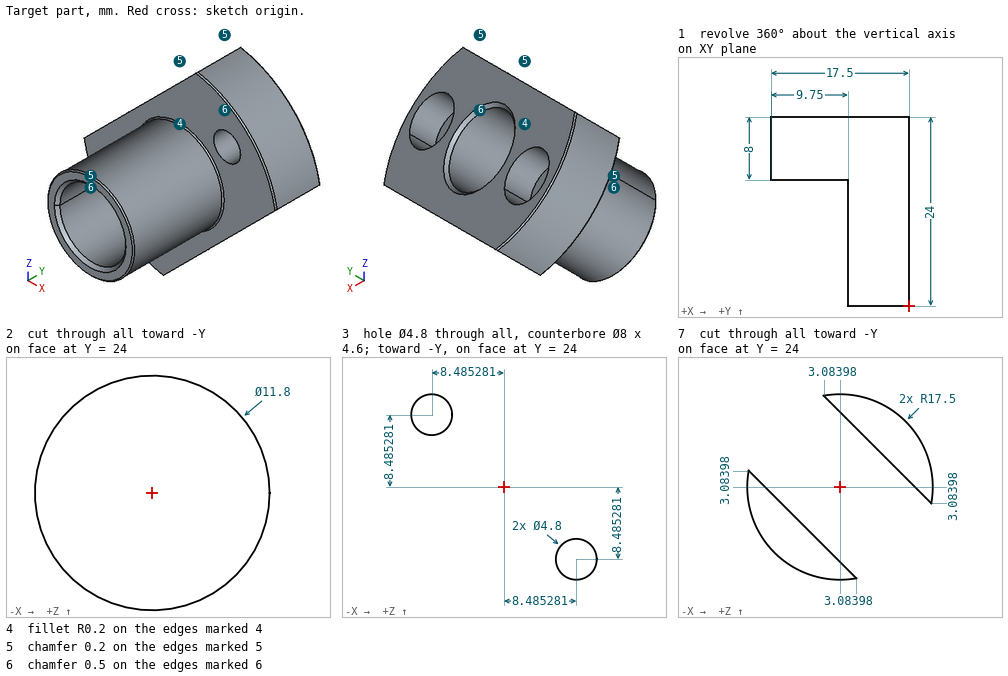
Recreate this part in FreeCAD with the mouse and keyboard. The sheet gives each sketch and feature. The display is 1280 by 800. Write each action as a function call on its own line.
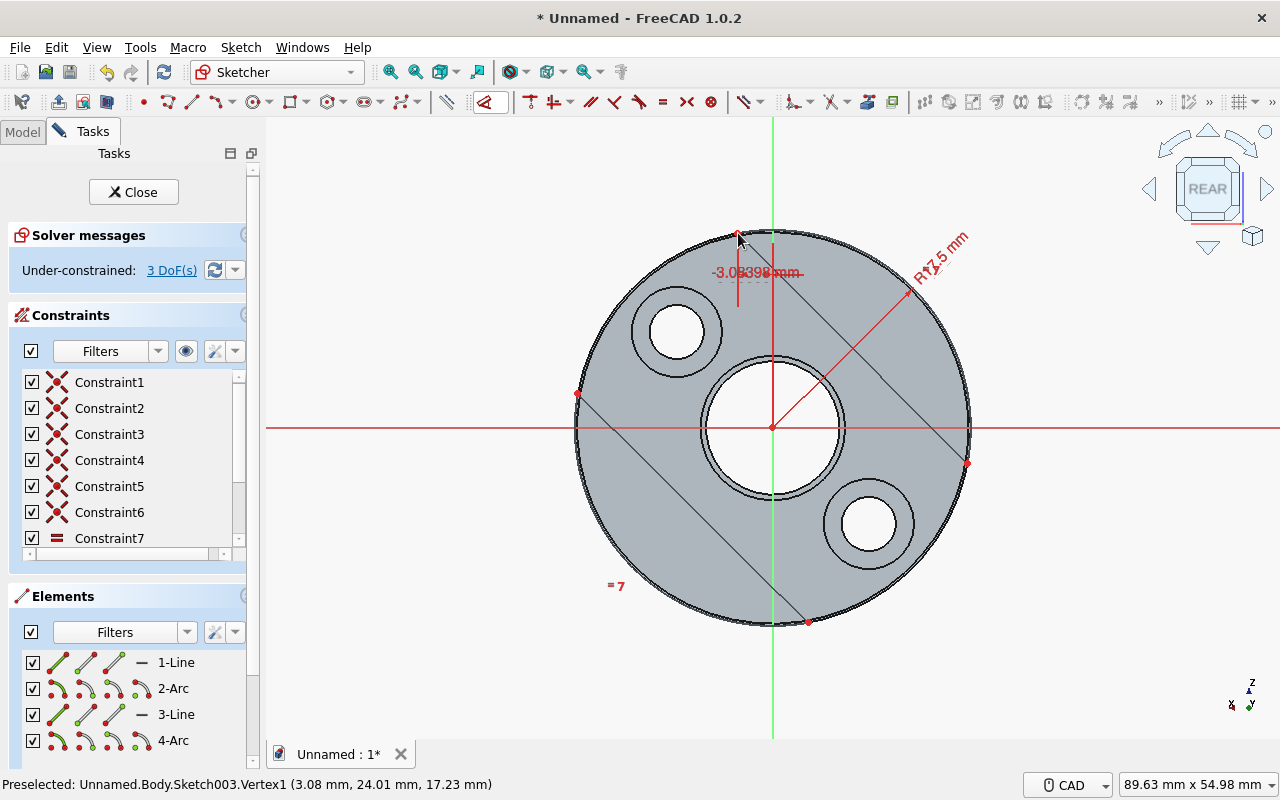
click(968, 464)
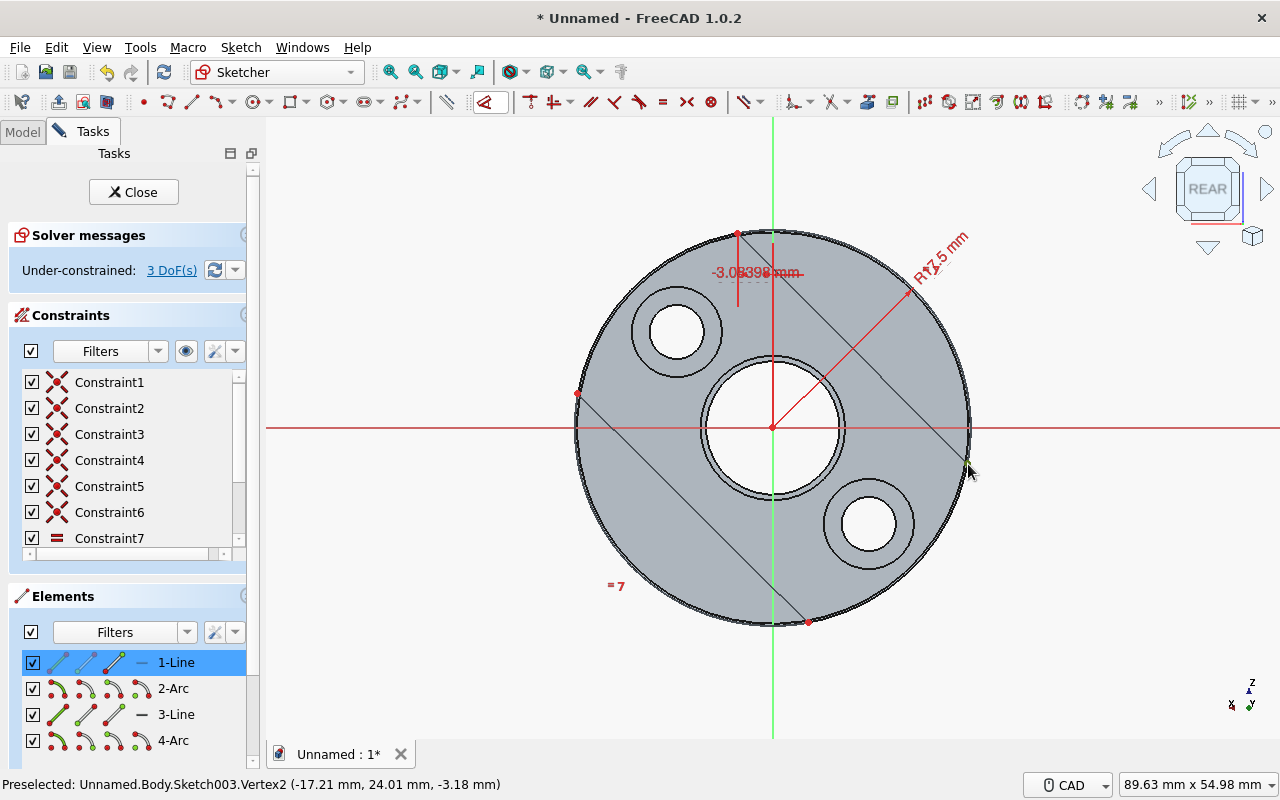
click(502, 102)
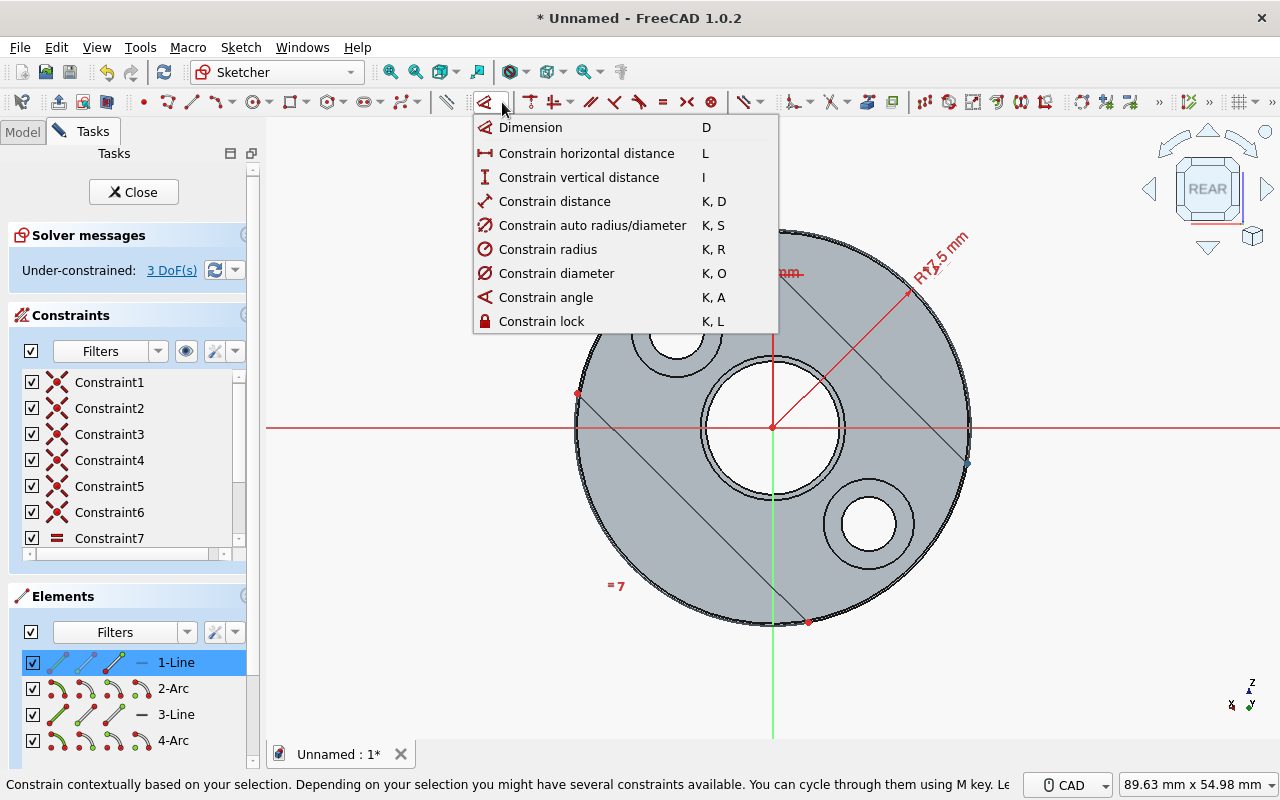
click(626, 177)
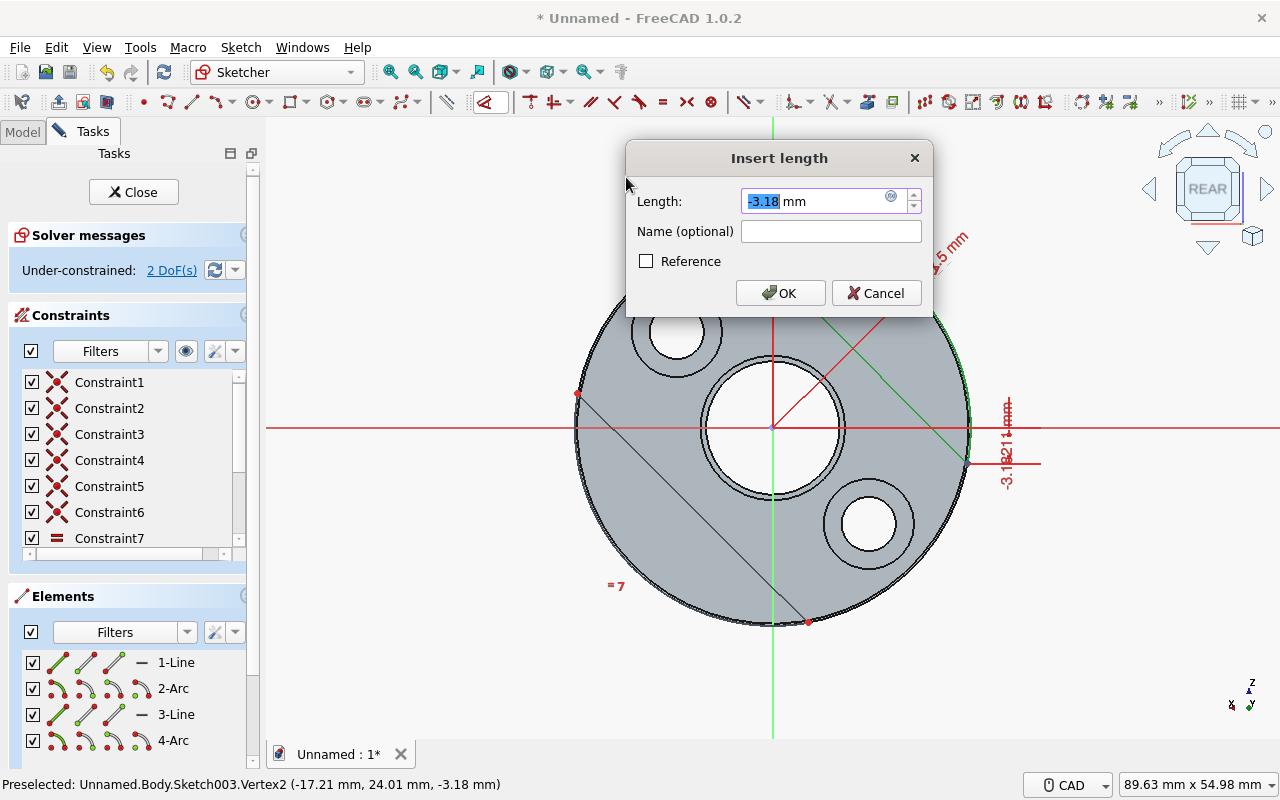
text(-3.08398)
key(Return)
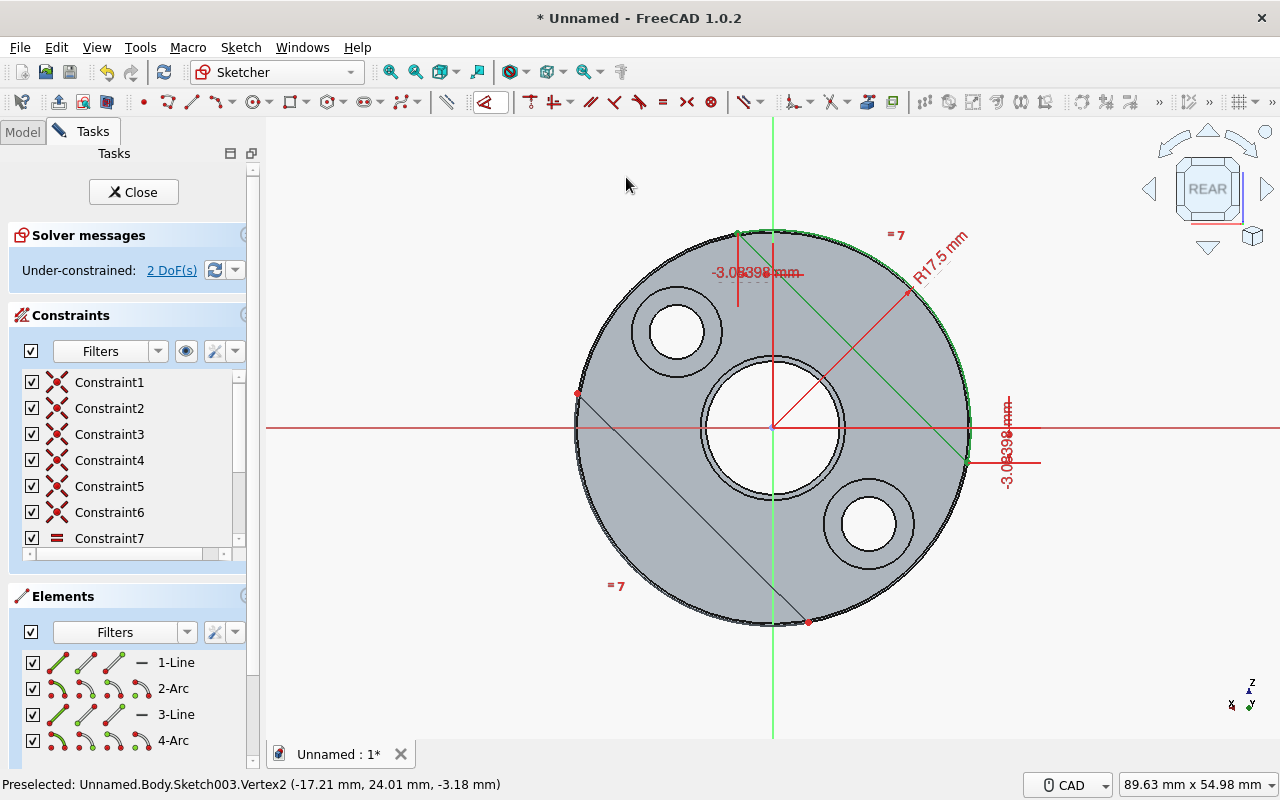
click(808, 623)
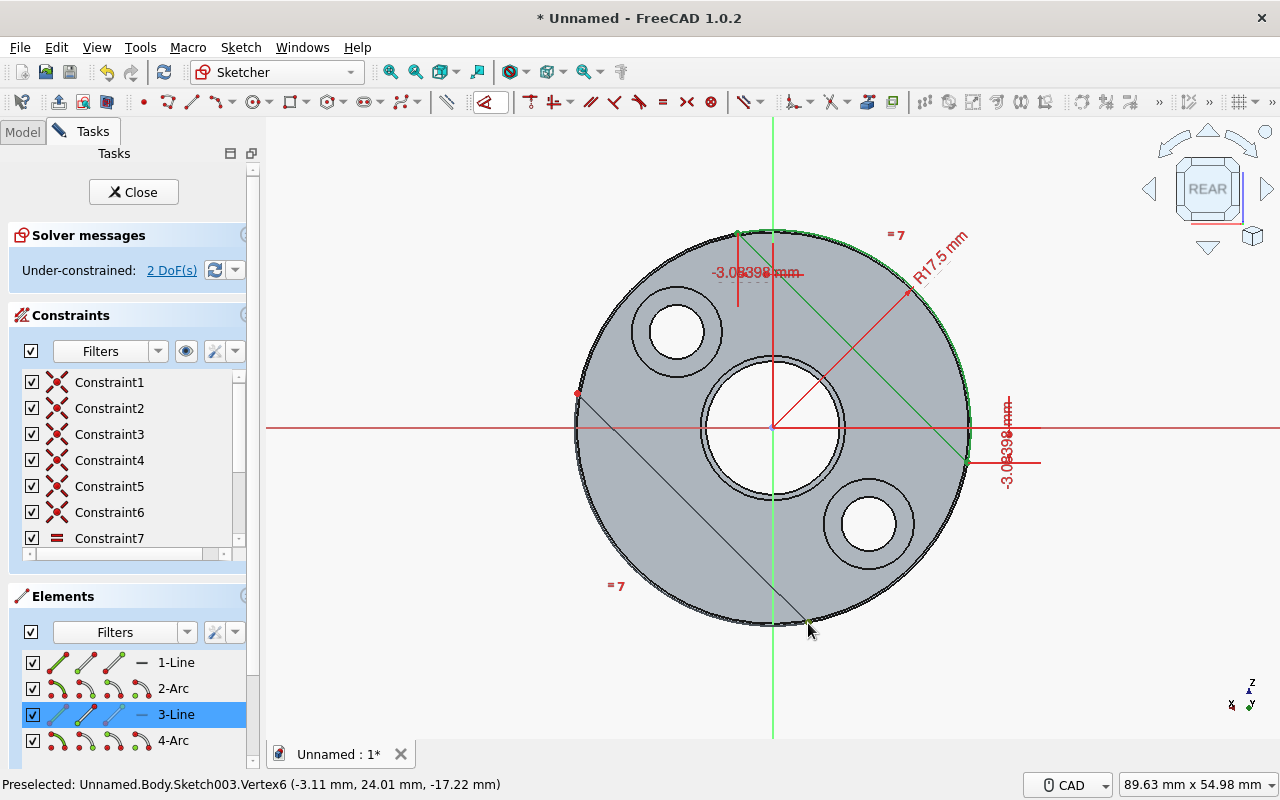
key(l)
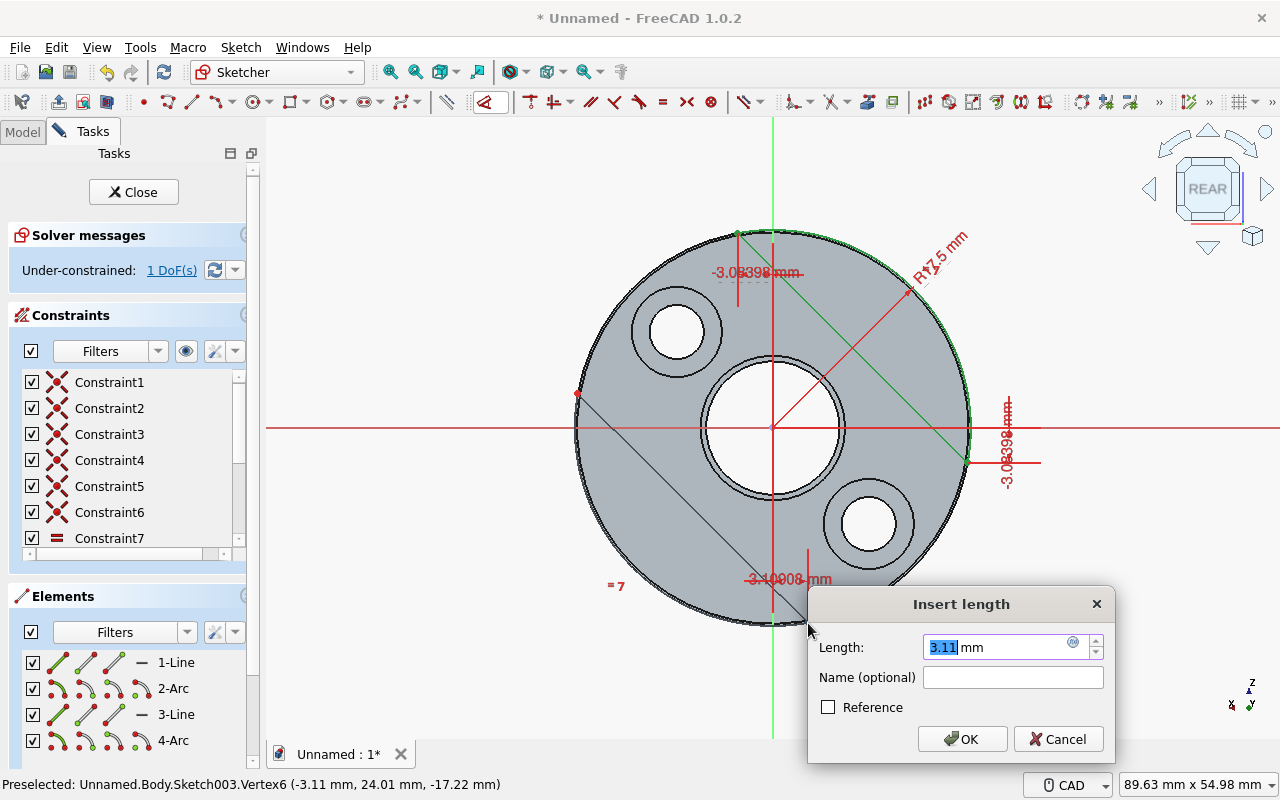
text(3.08398)
key(Return)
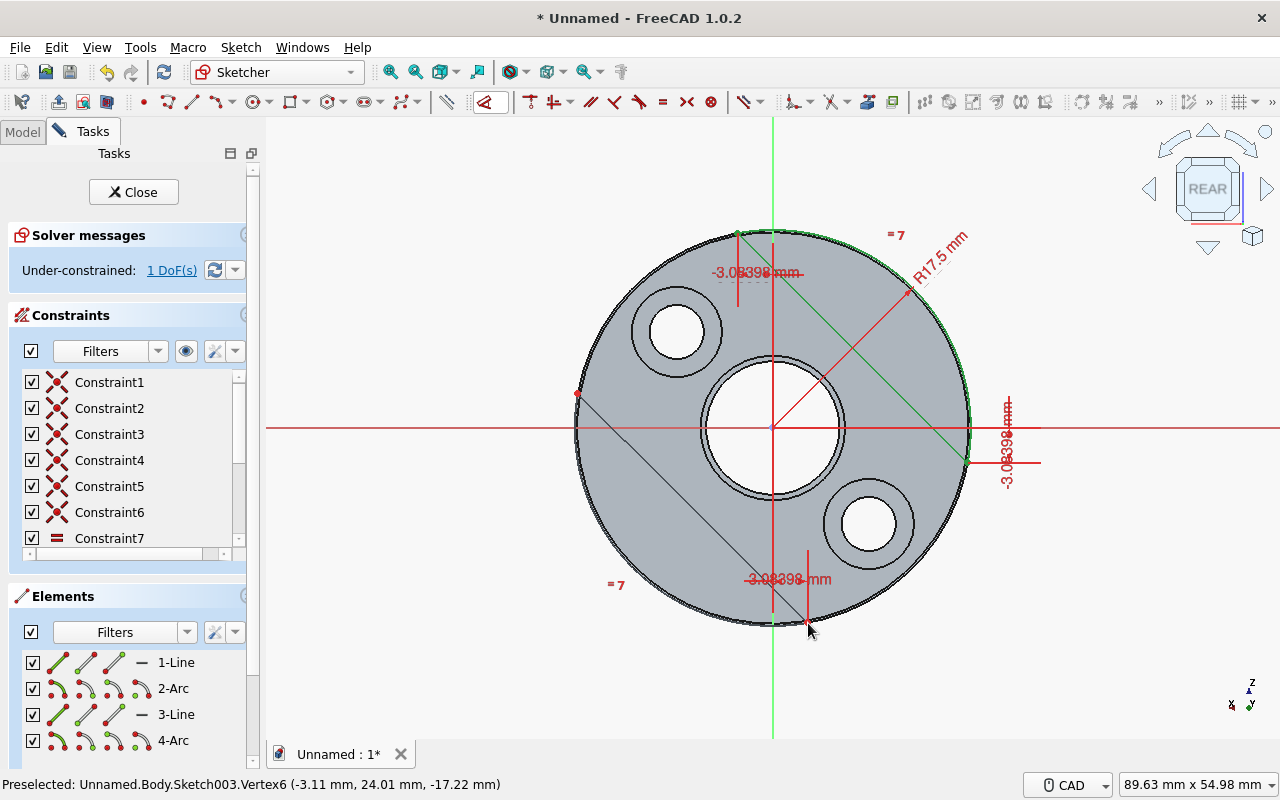
click(578, 394)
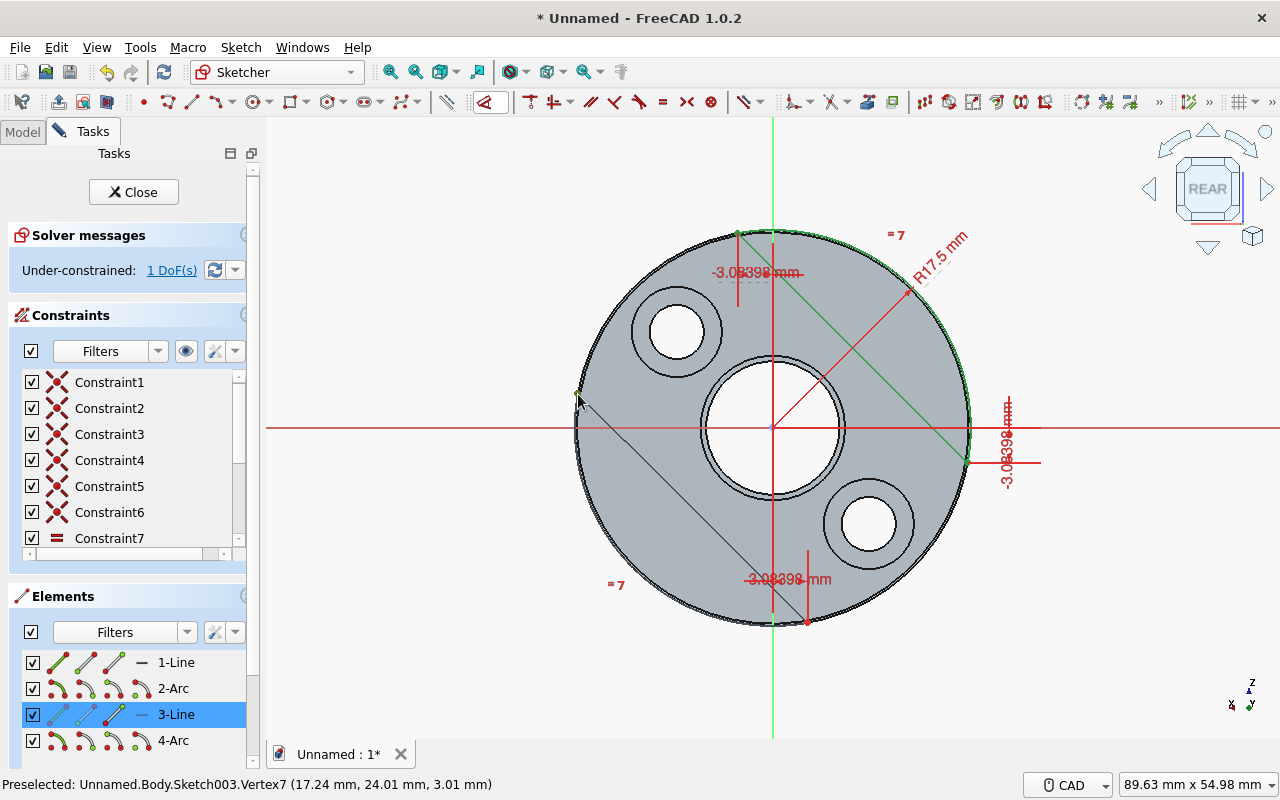
click(502, 102)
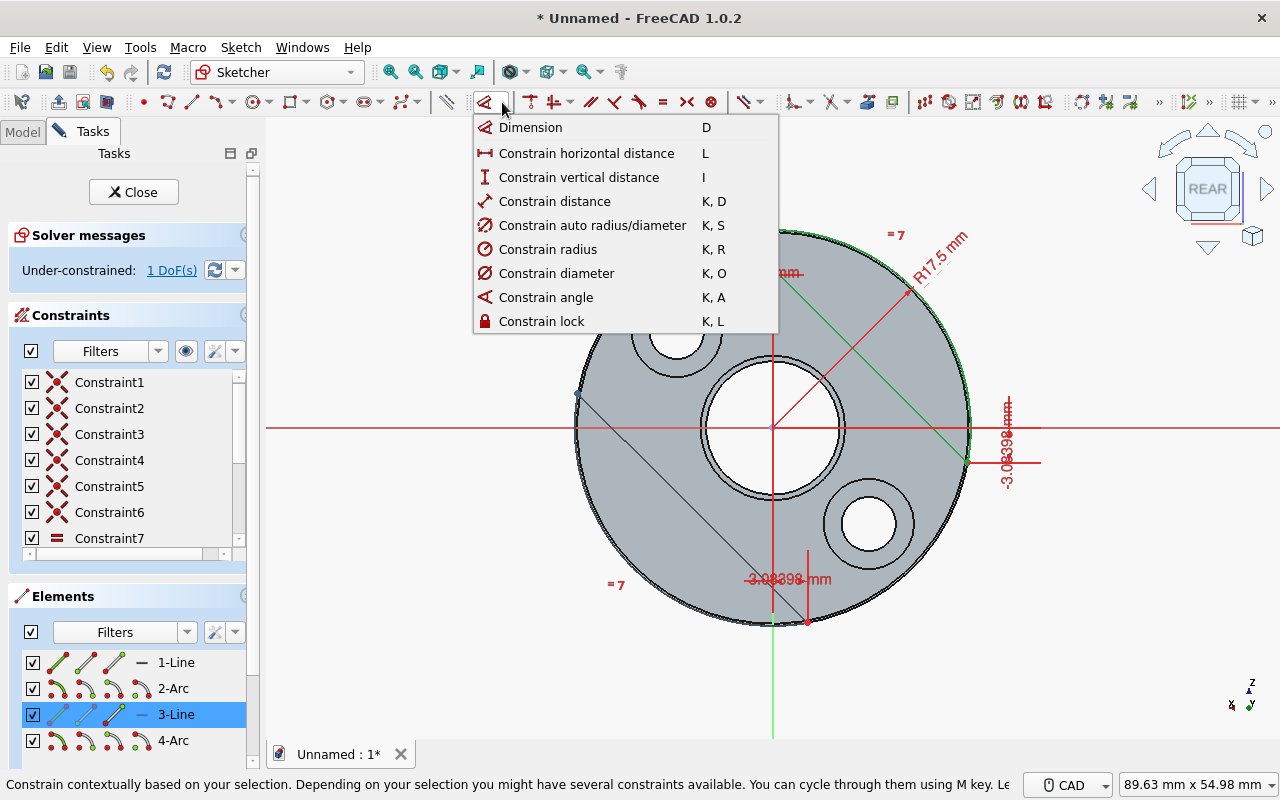
click(626, 177)